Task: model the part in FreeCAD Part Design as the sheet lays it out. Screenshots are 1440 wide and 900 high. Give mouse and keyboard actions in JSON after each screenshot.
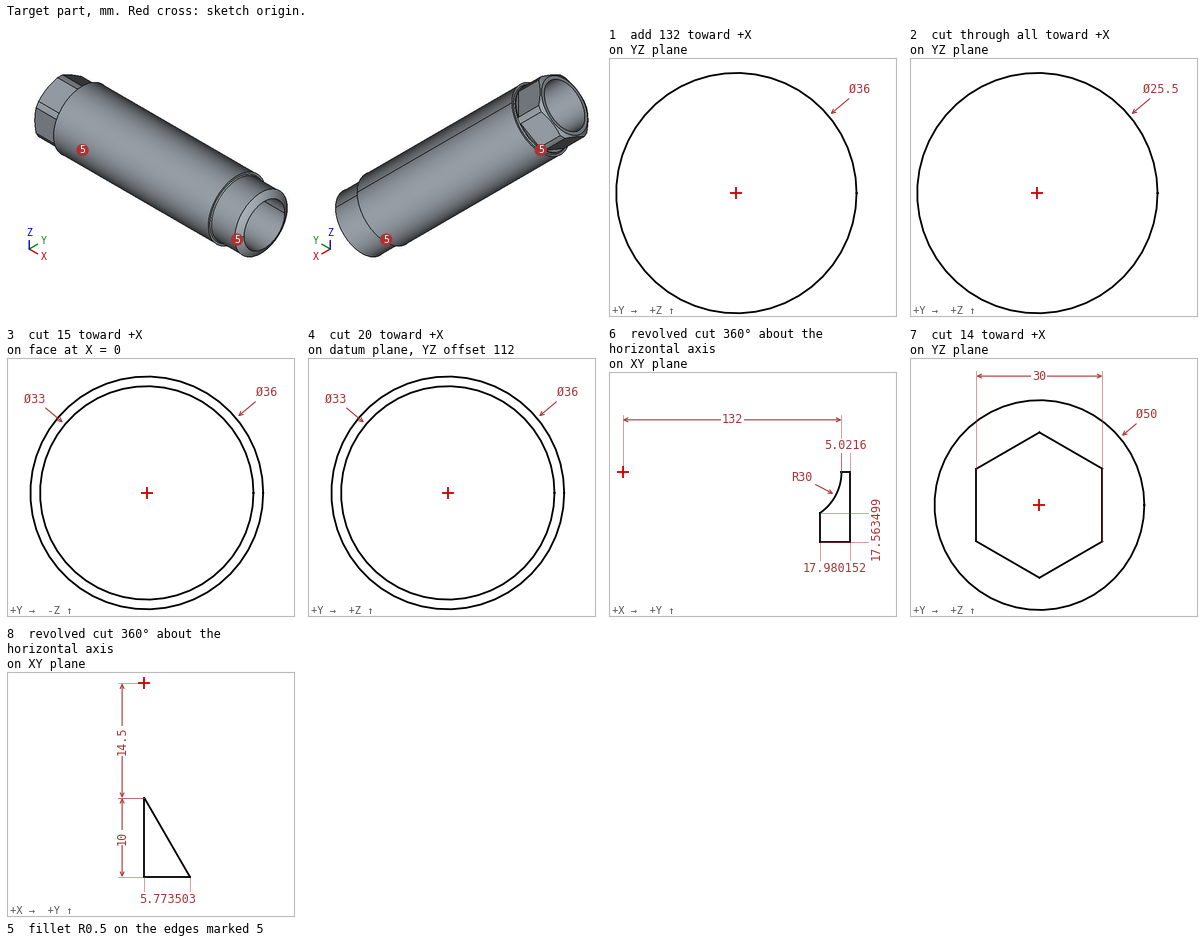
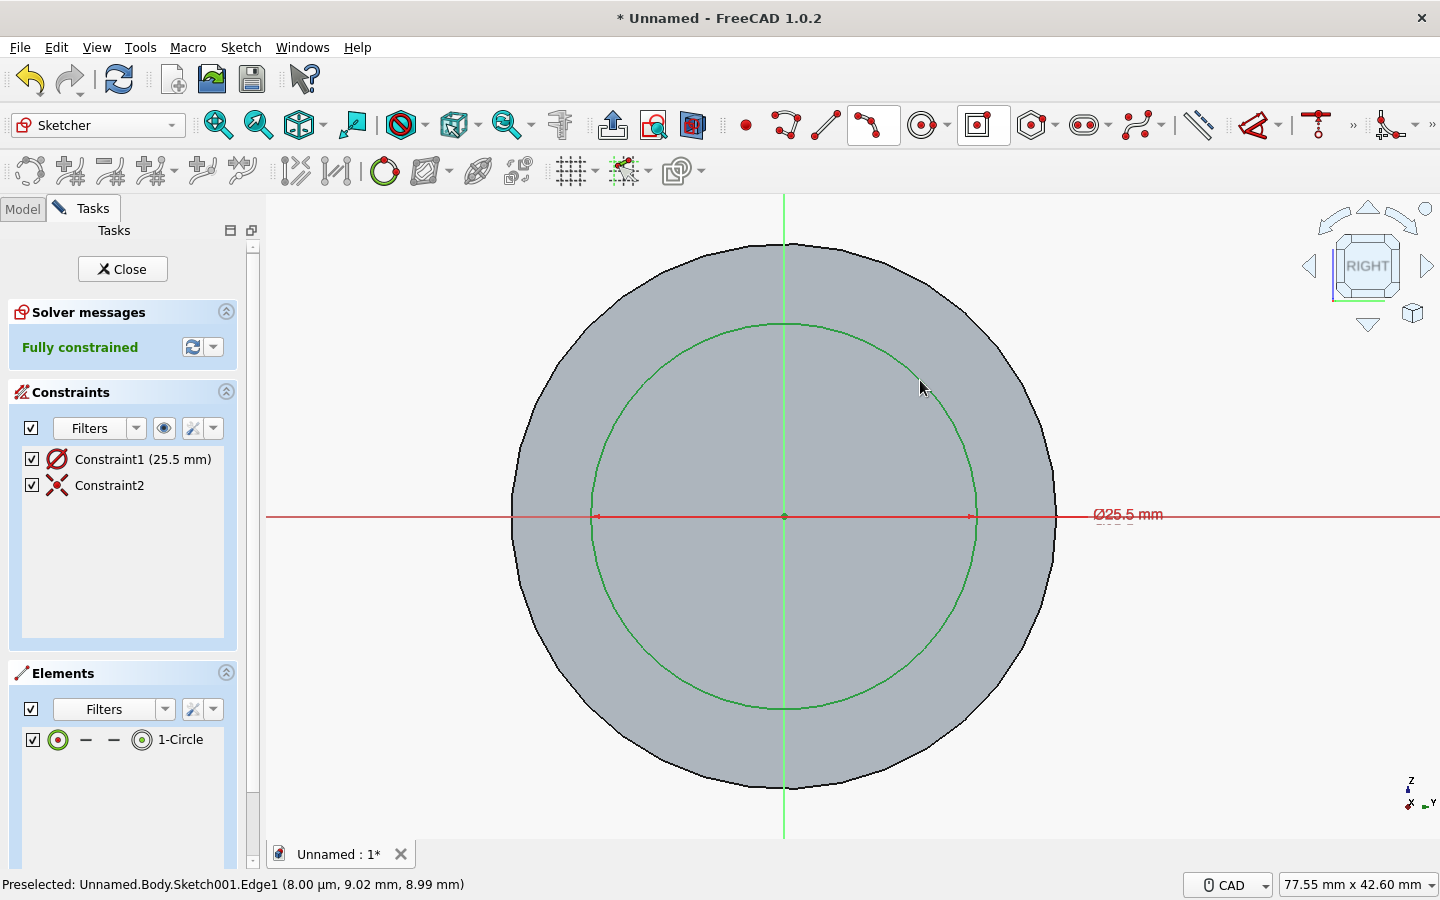
{"action": "left_click", "coordinate": [123, 269]}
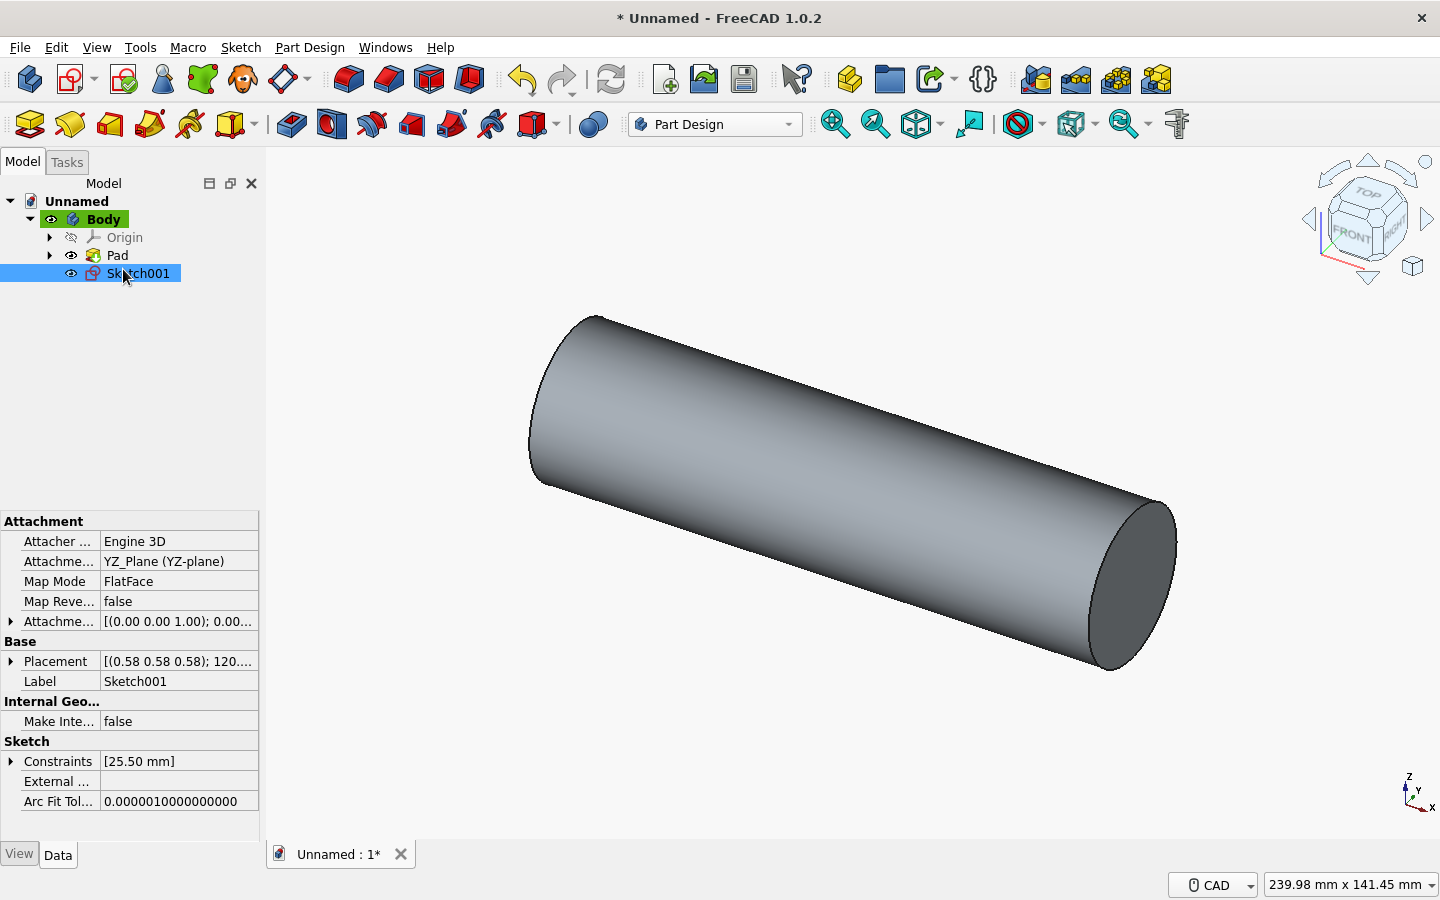
{"action": "left_click", "coordinate": [292, 124]}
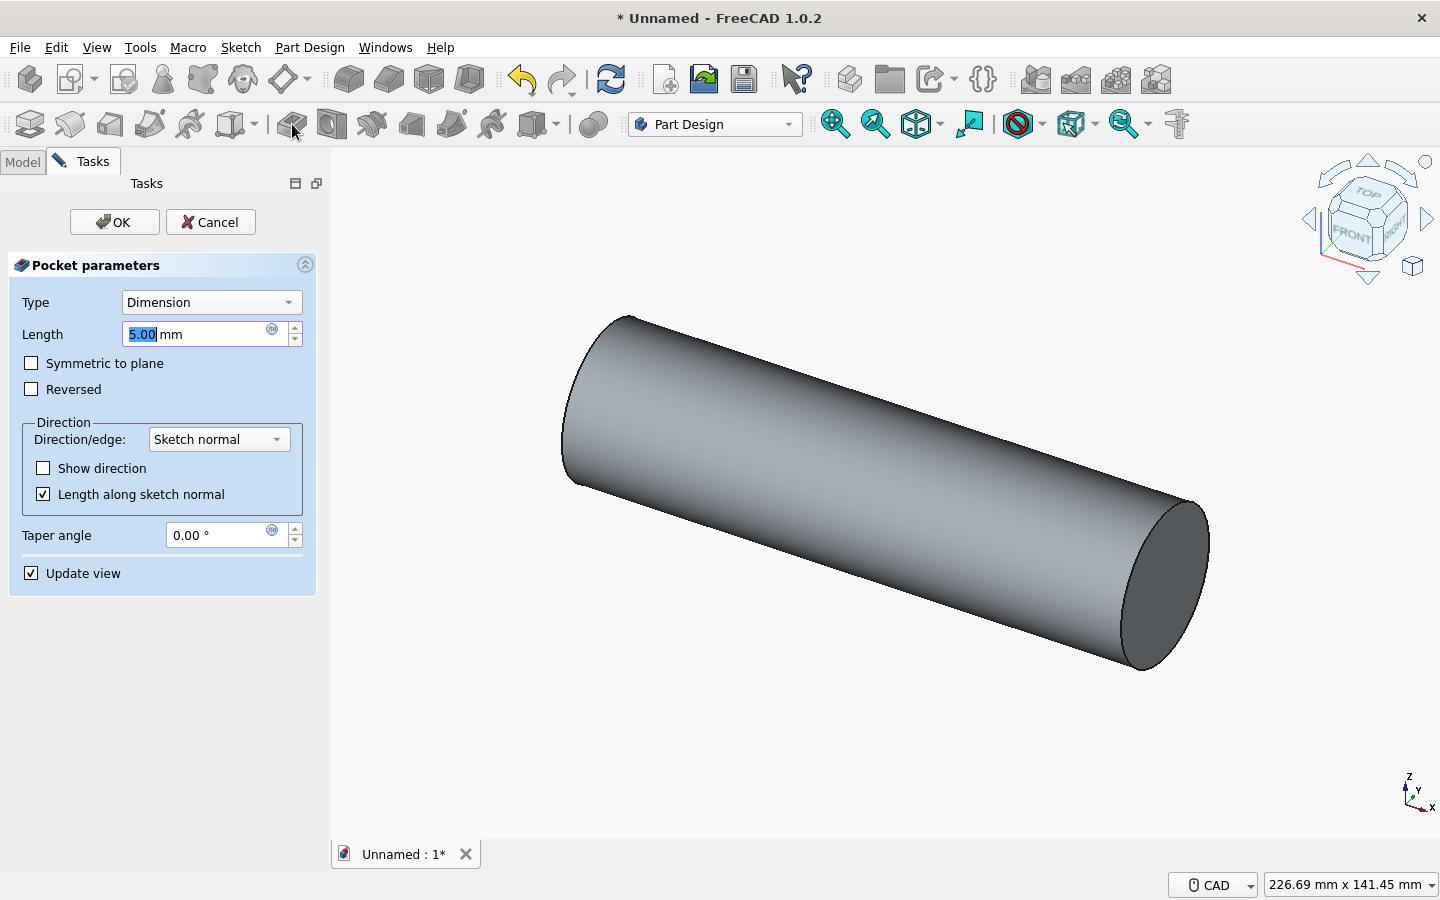
{"action": "left_click", "coordinate": [212, 302]}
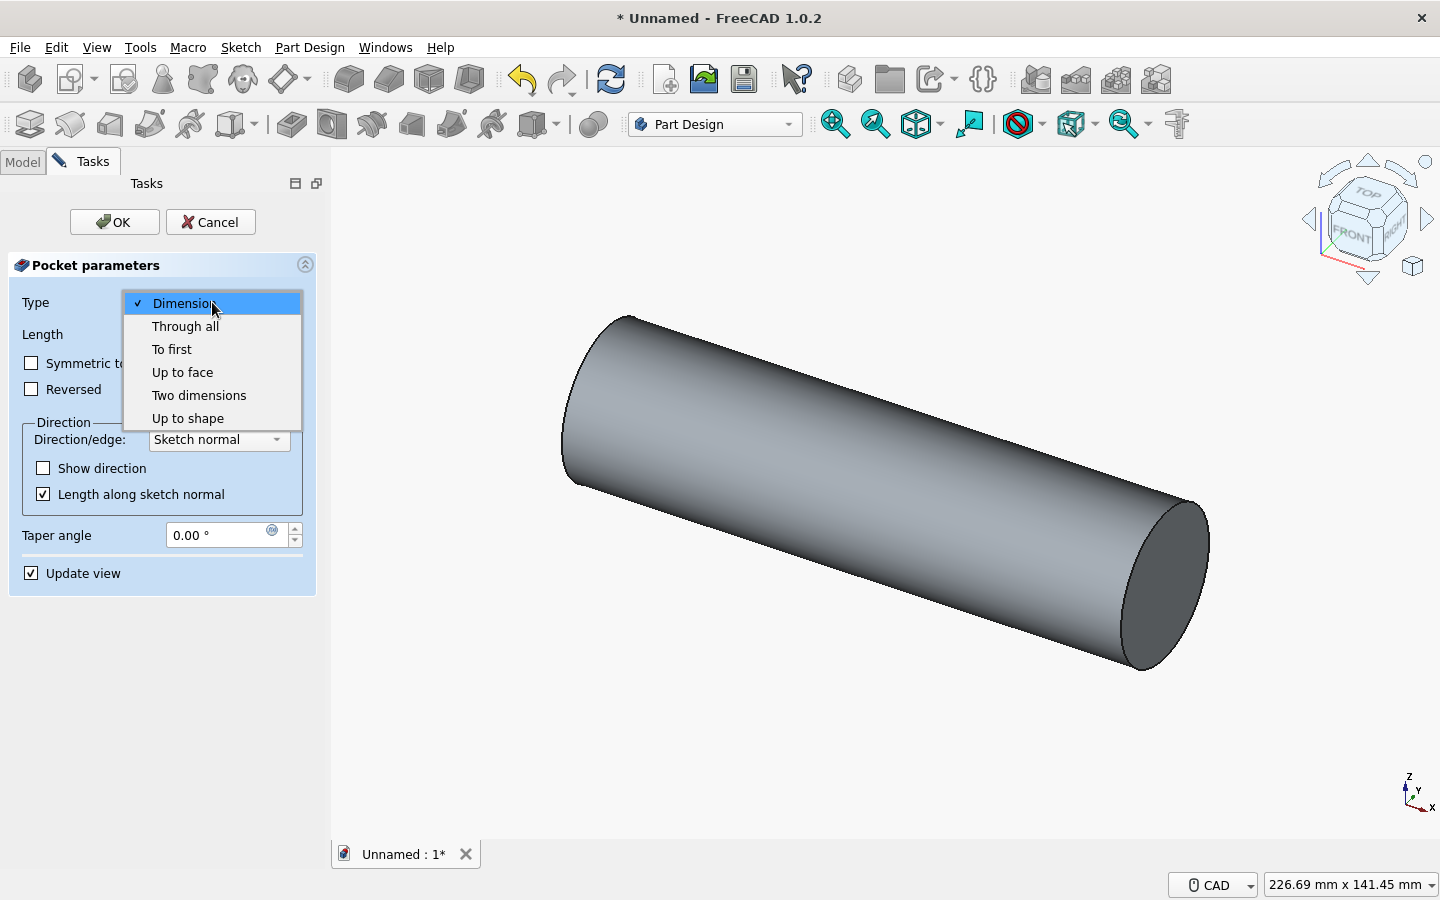
{"action": "left_click", "coordinate": [212, 326]}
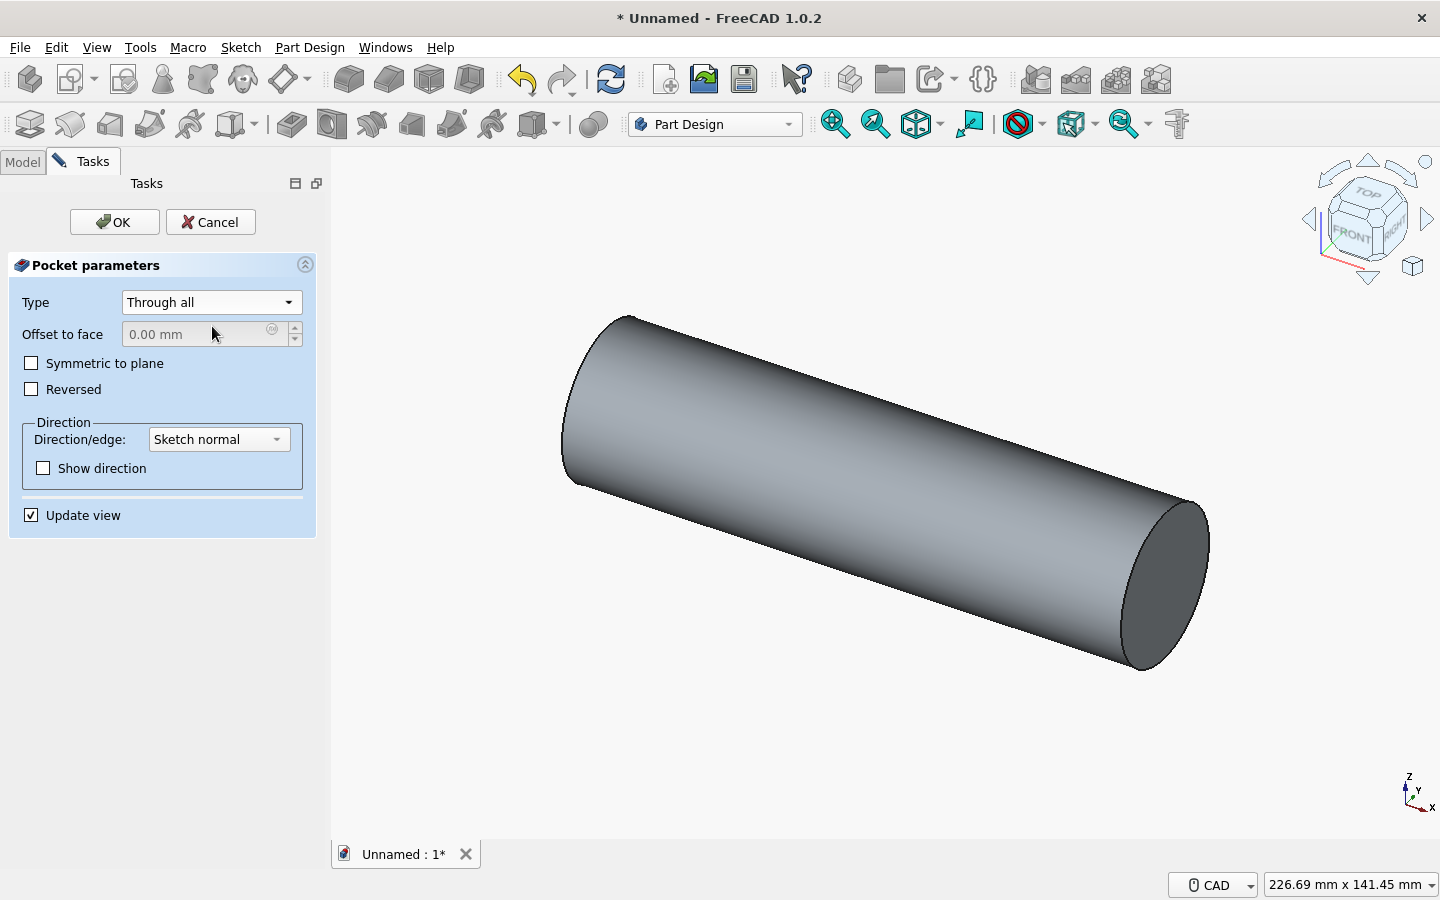
{"action": "left_click", "coordinate": [30, 389]}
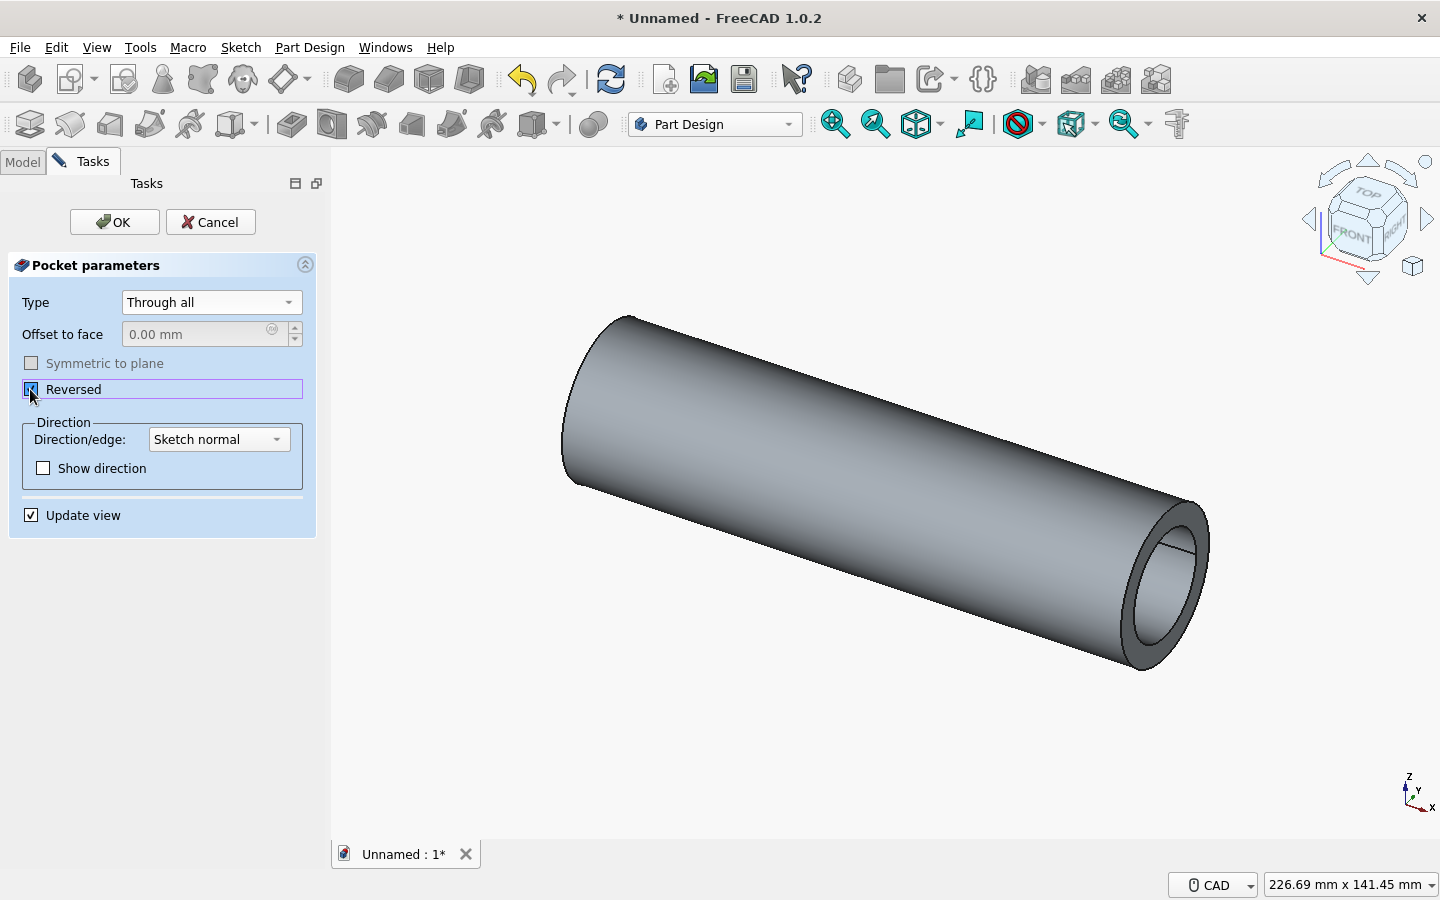
{"action": "left_click", "coordinate": [115, 222]}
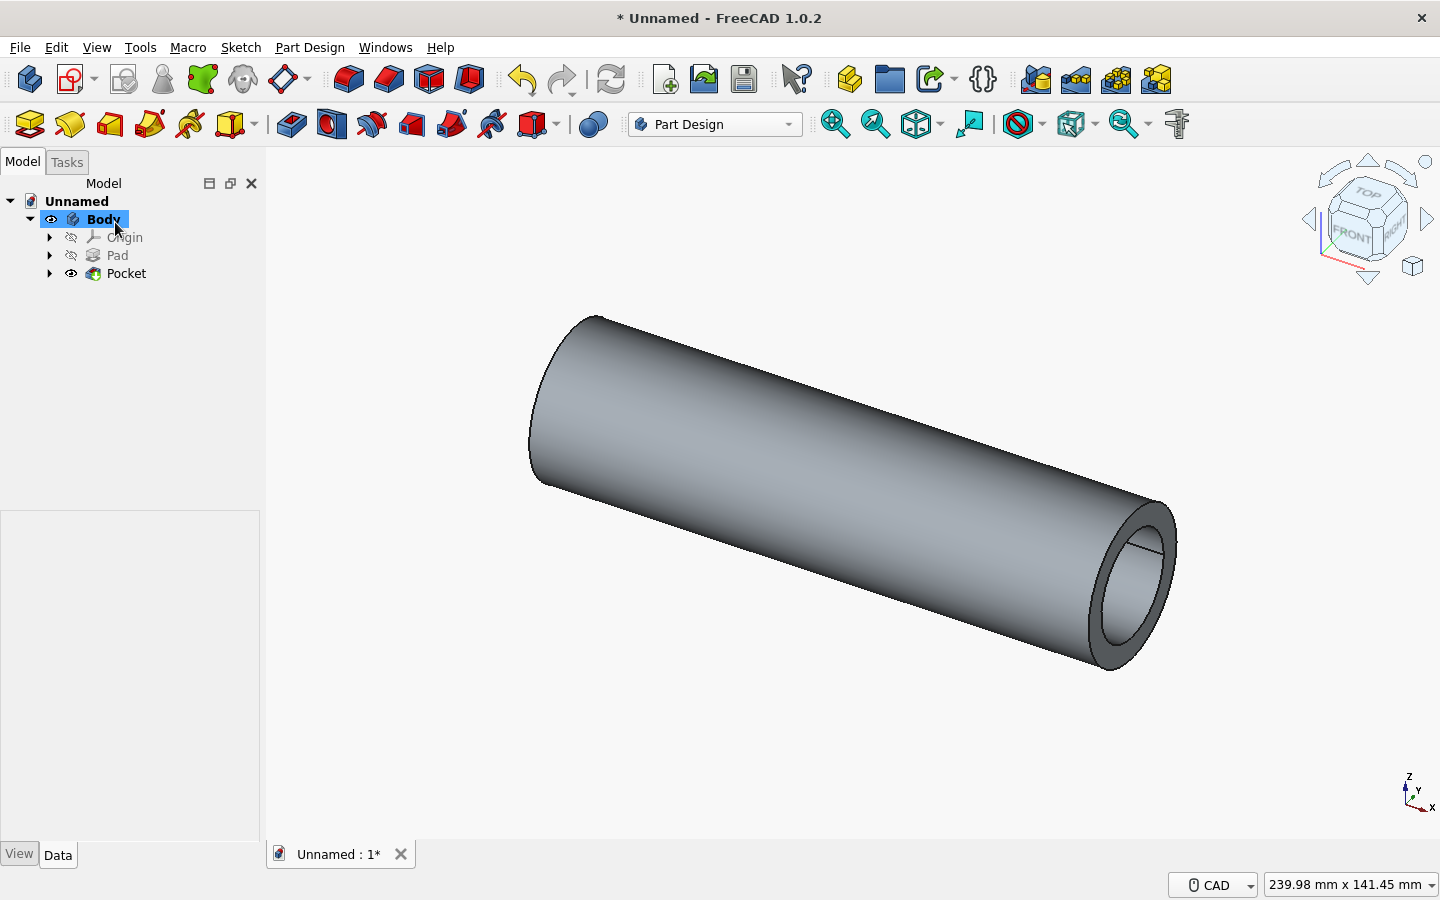
{"action": "key", "text": "6"}